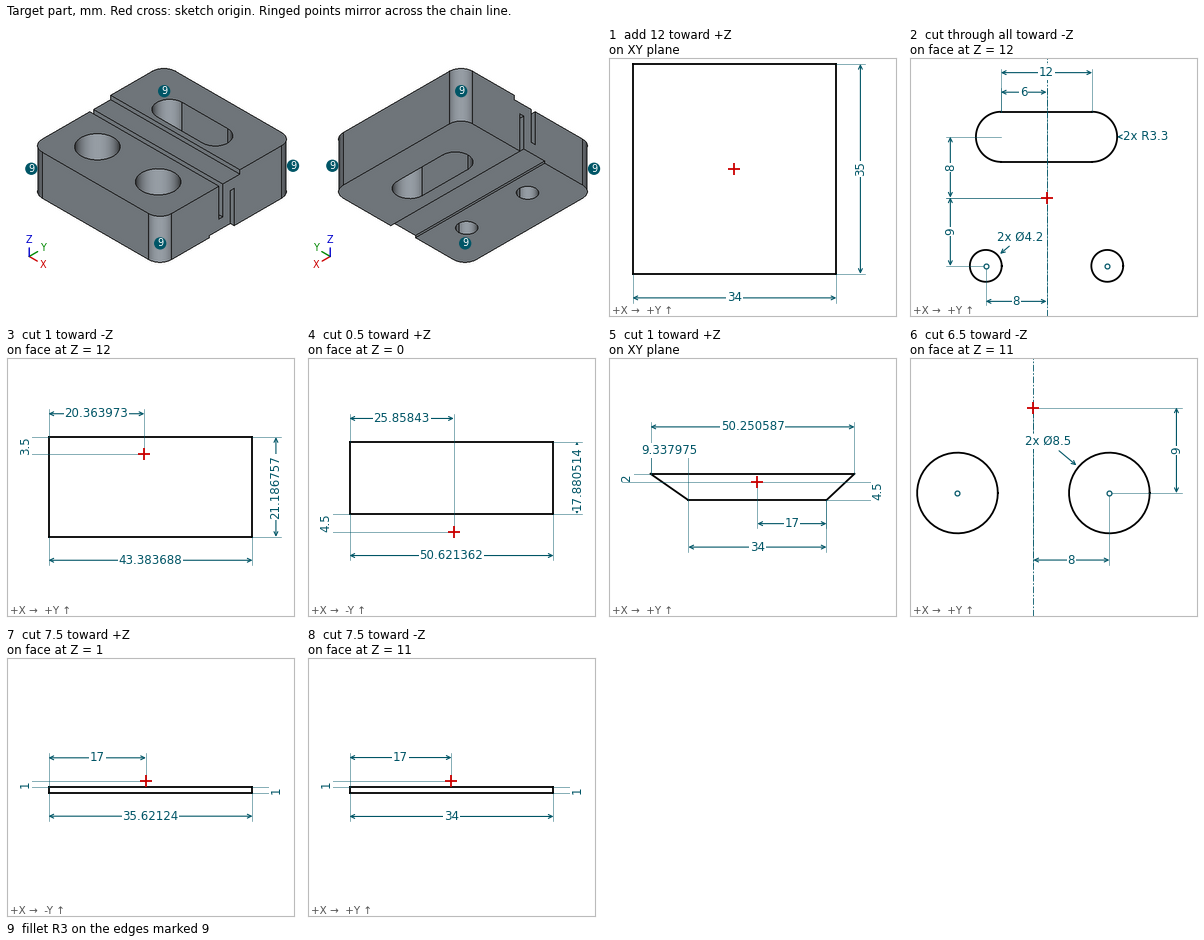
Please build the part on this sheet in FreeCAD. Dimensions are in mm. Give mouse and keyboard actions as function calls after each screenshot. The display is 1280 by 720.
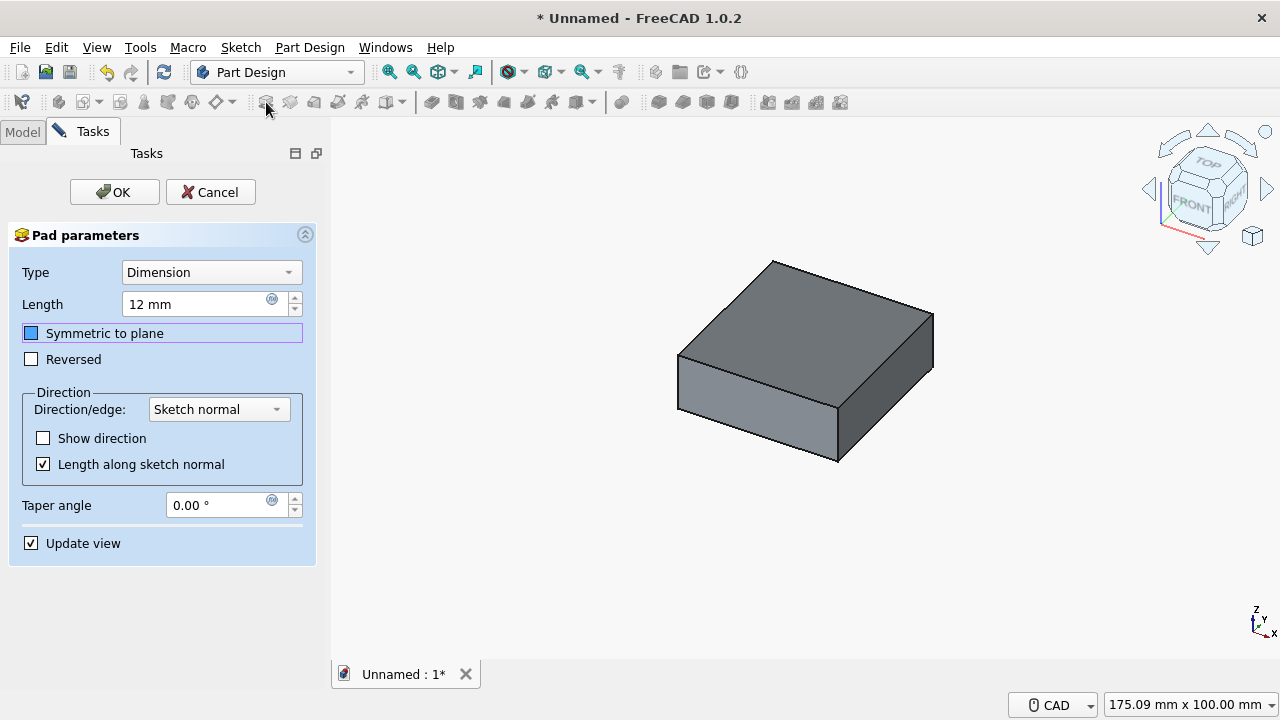
click(115, 192)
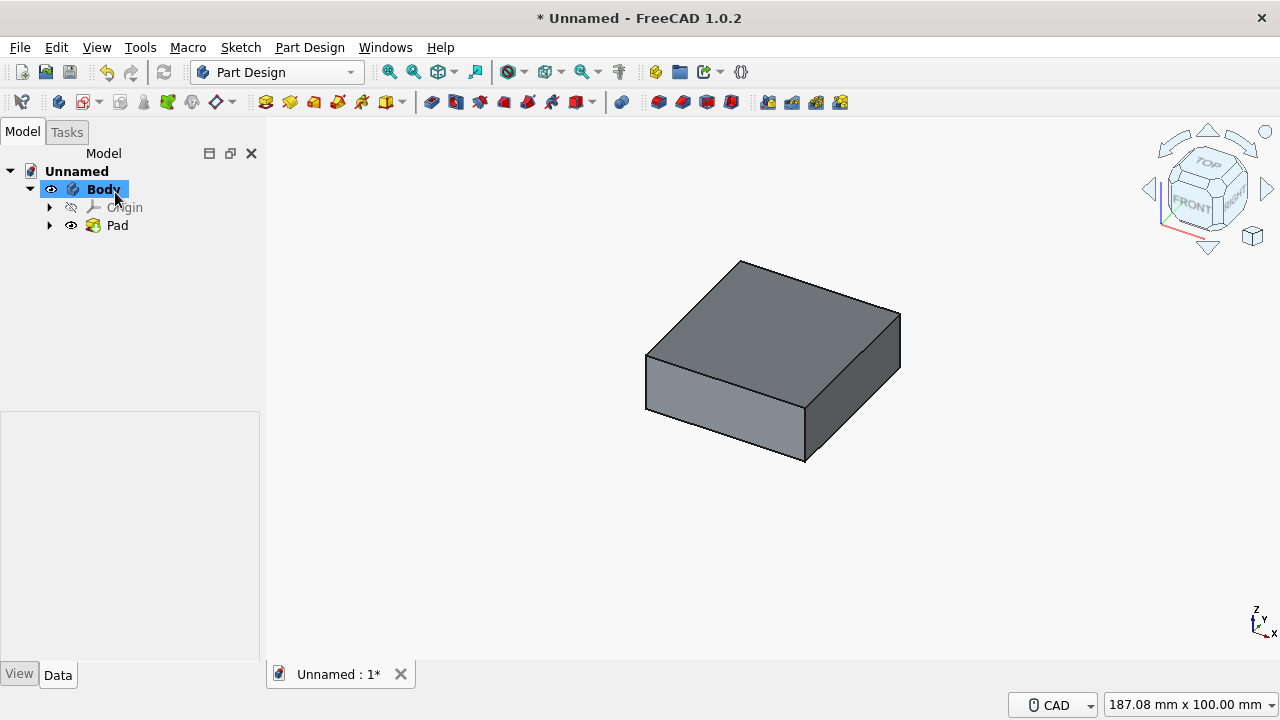
key(v)
key(f)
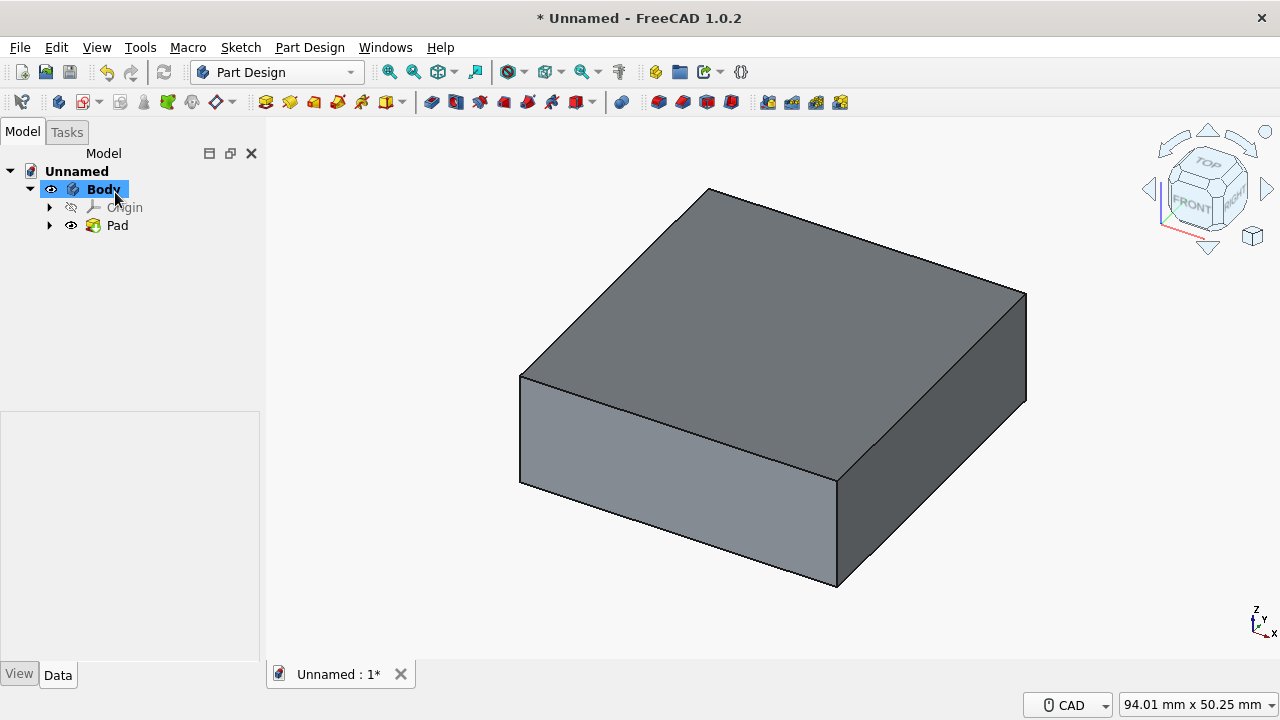
click(773, 334)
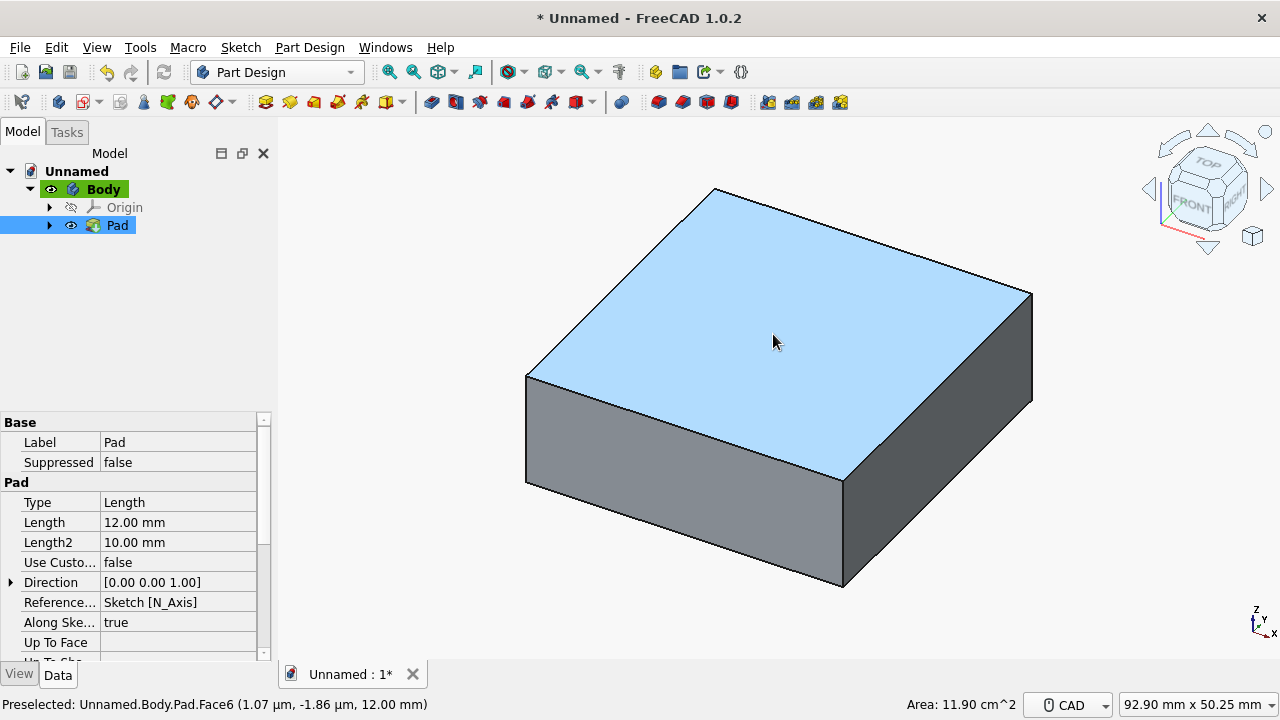
click(84, 102)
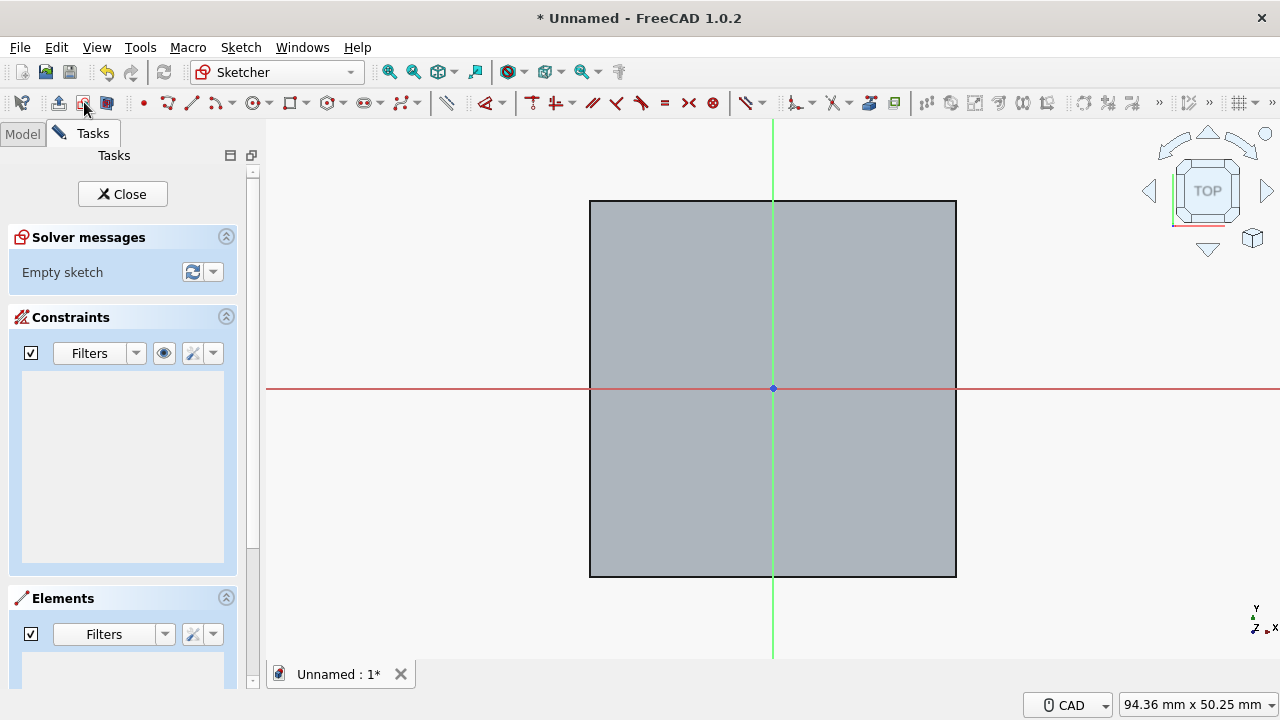
scroll(912, 386, up, 2)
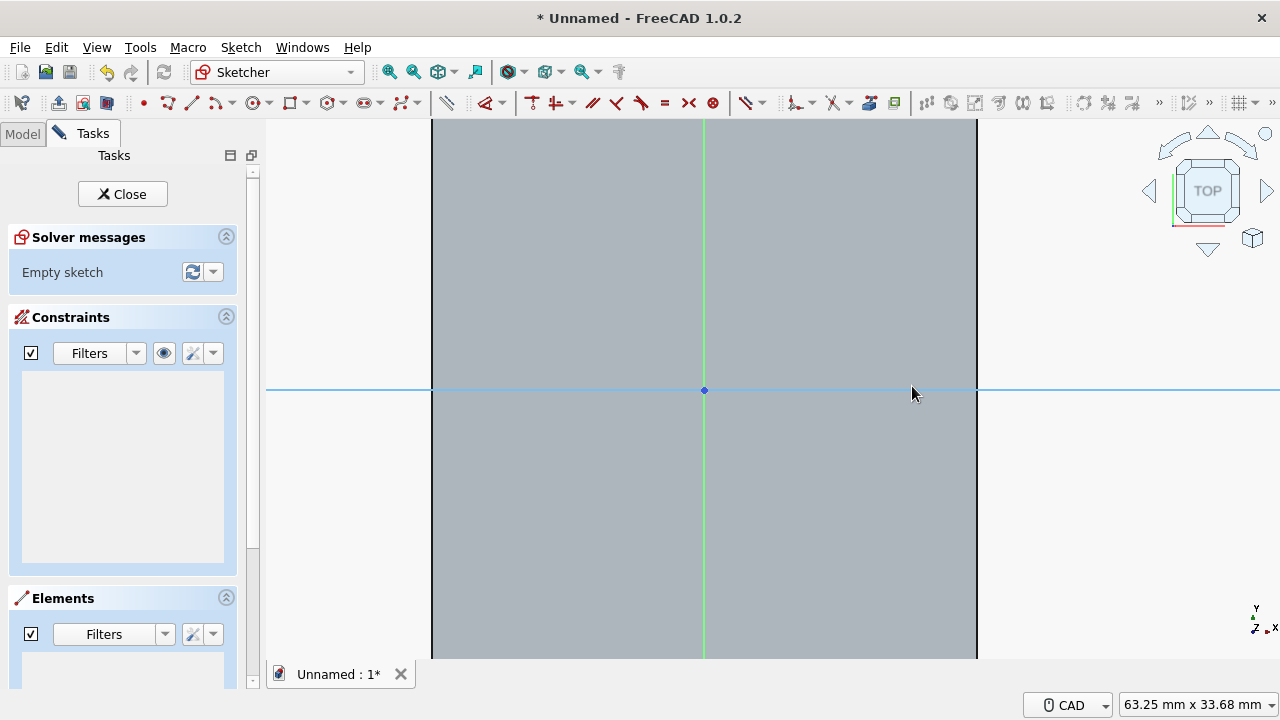
key(g)
key(s)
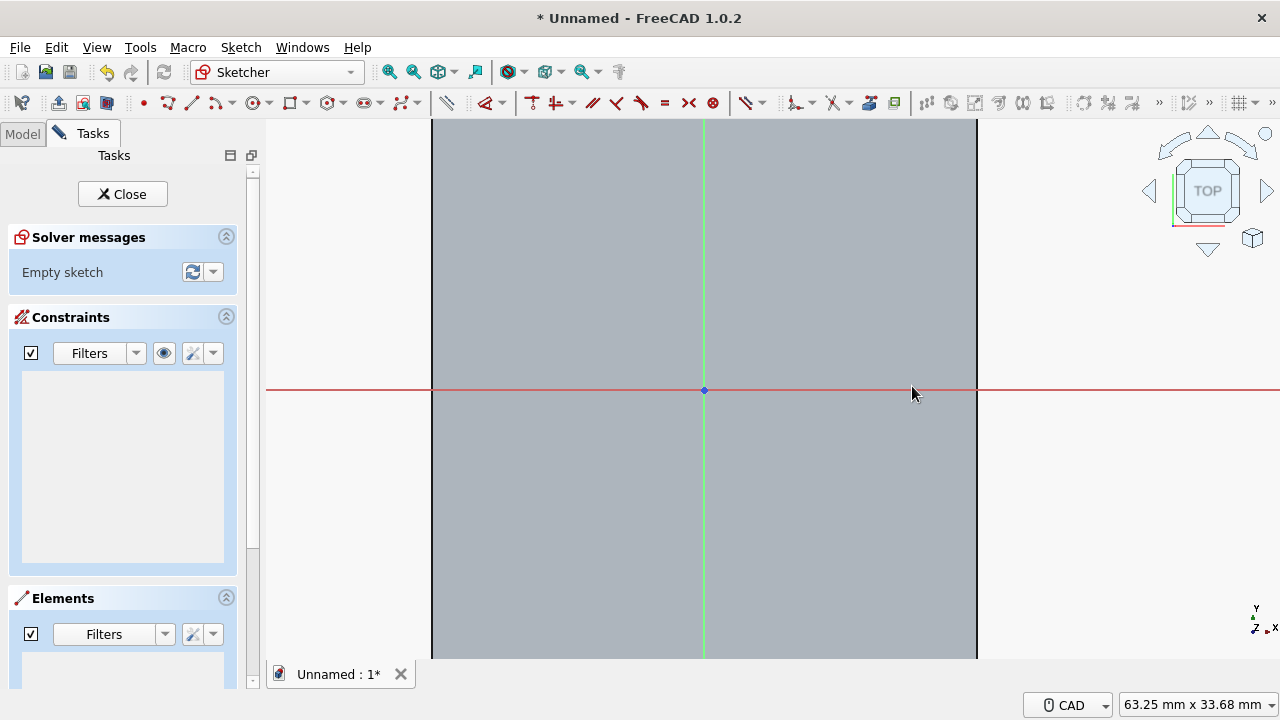
click(608, 262)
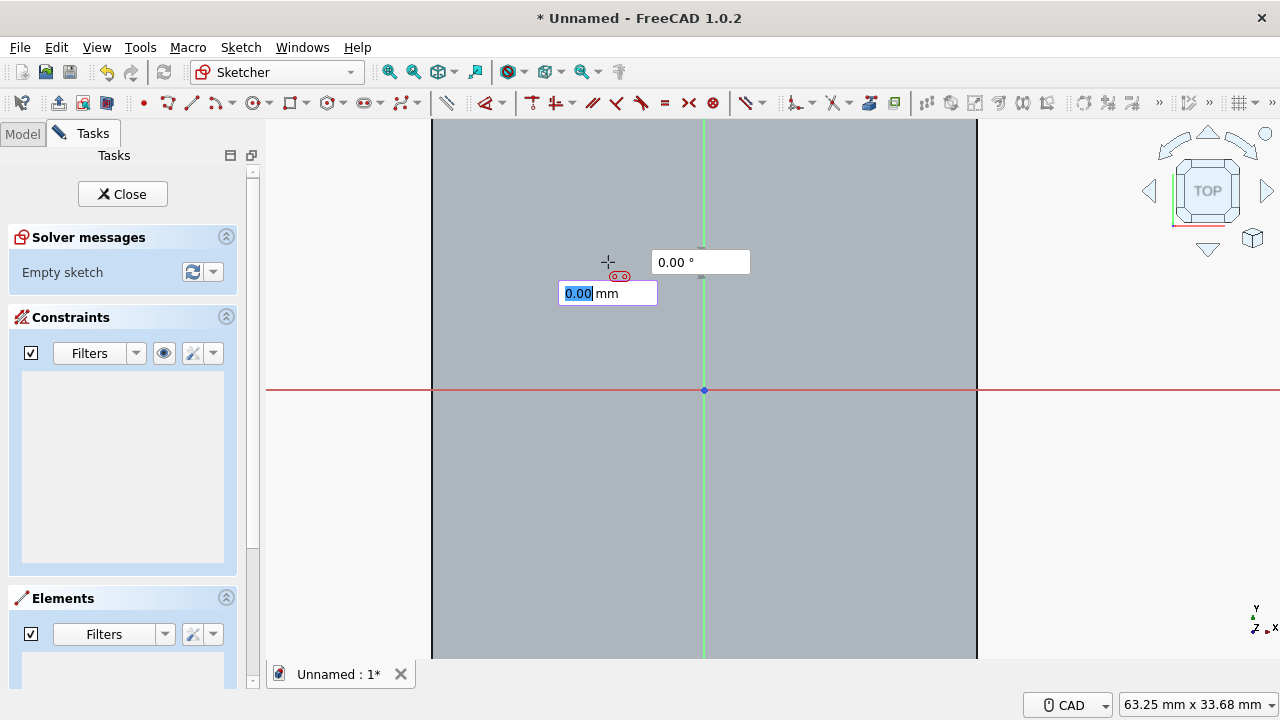
click(801, 262)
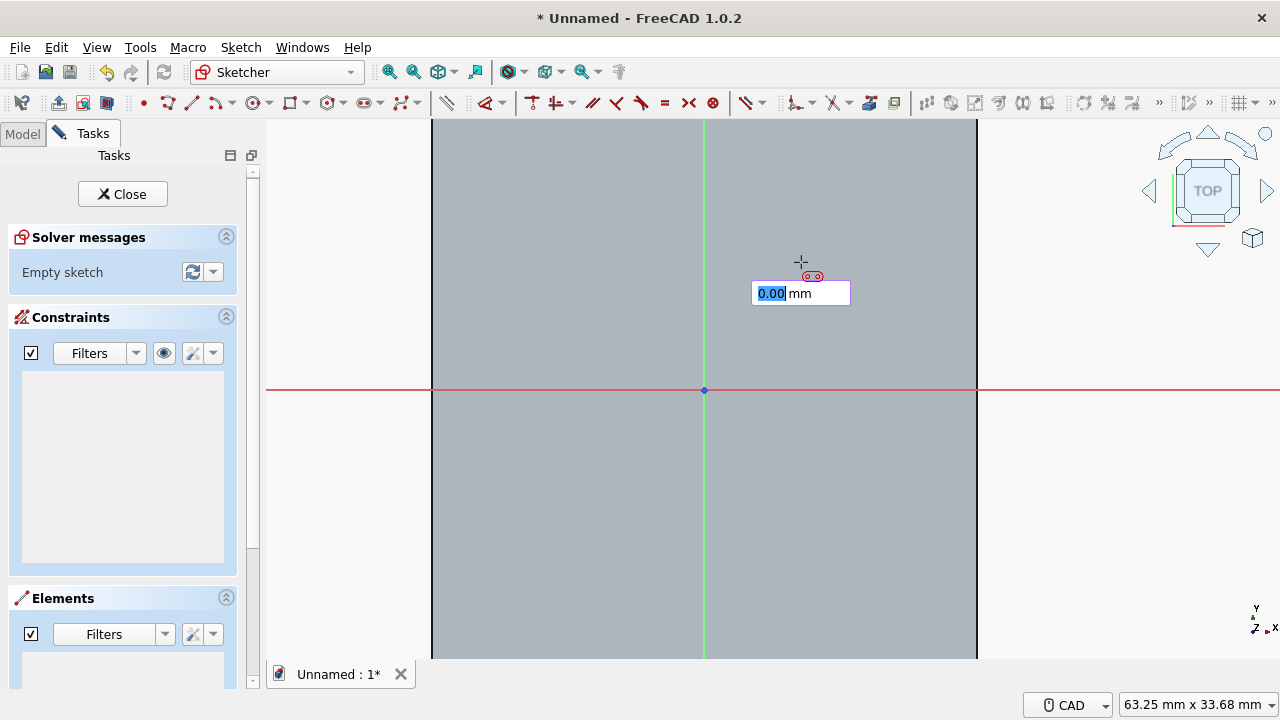
click(733, 209)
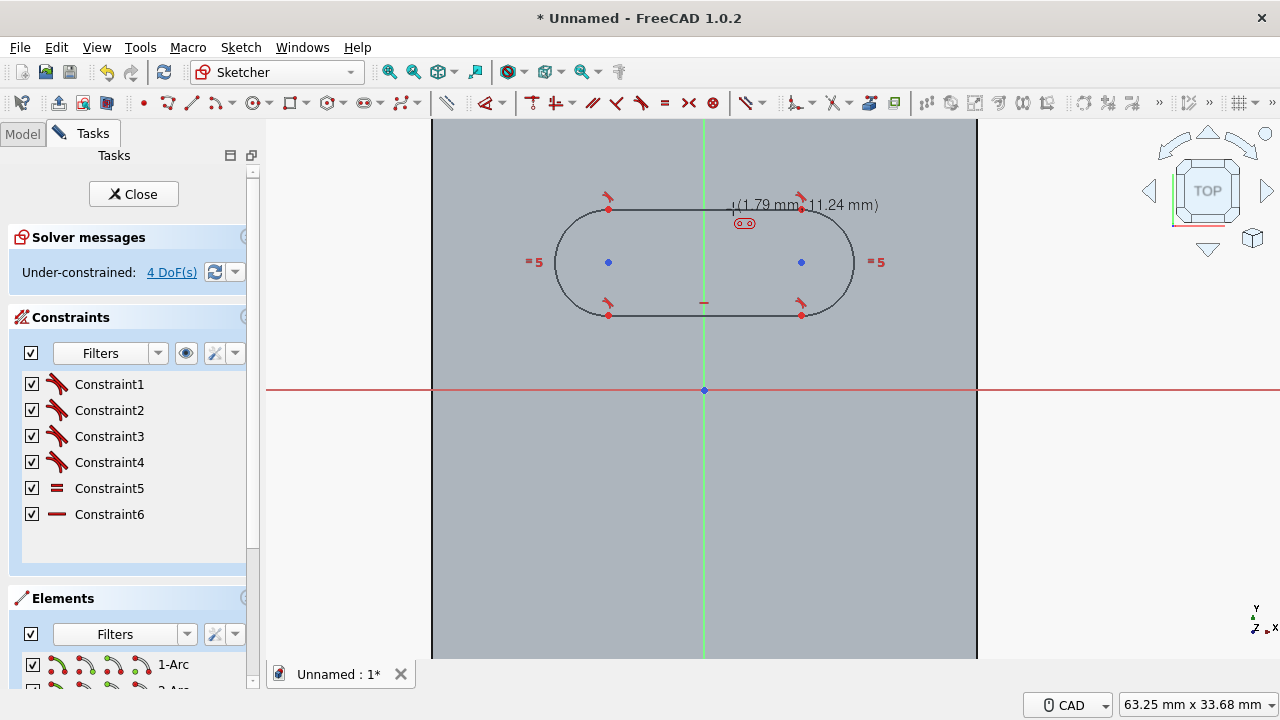
key(g)
key(c)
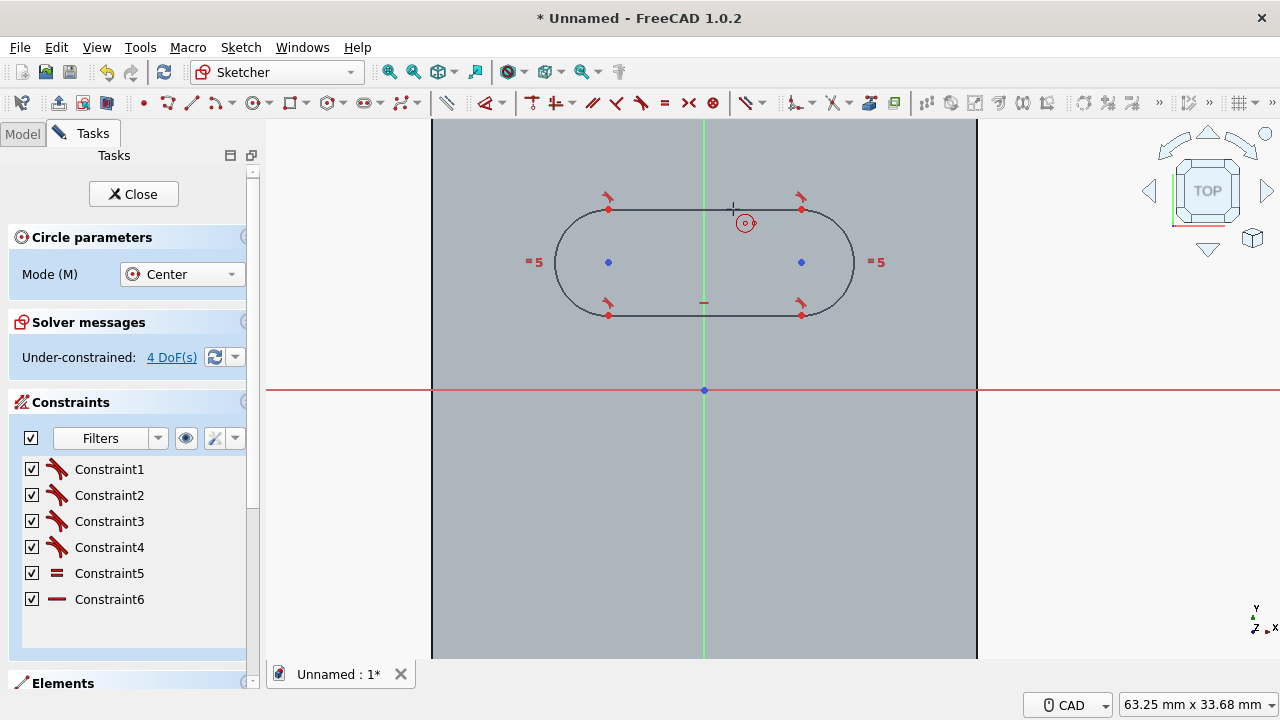
click(576, 535)
move(600, 511)